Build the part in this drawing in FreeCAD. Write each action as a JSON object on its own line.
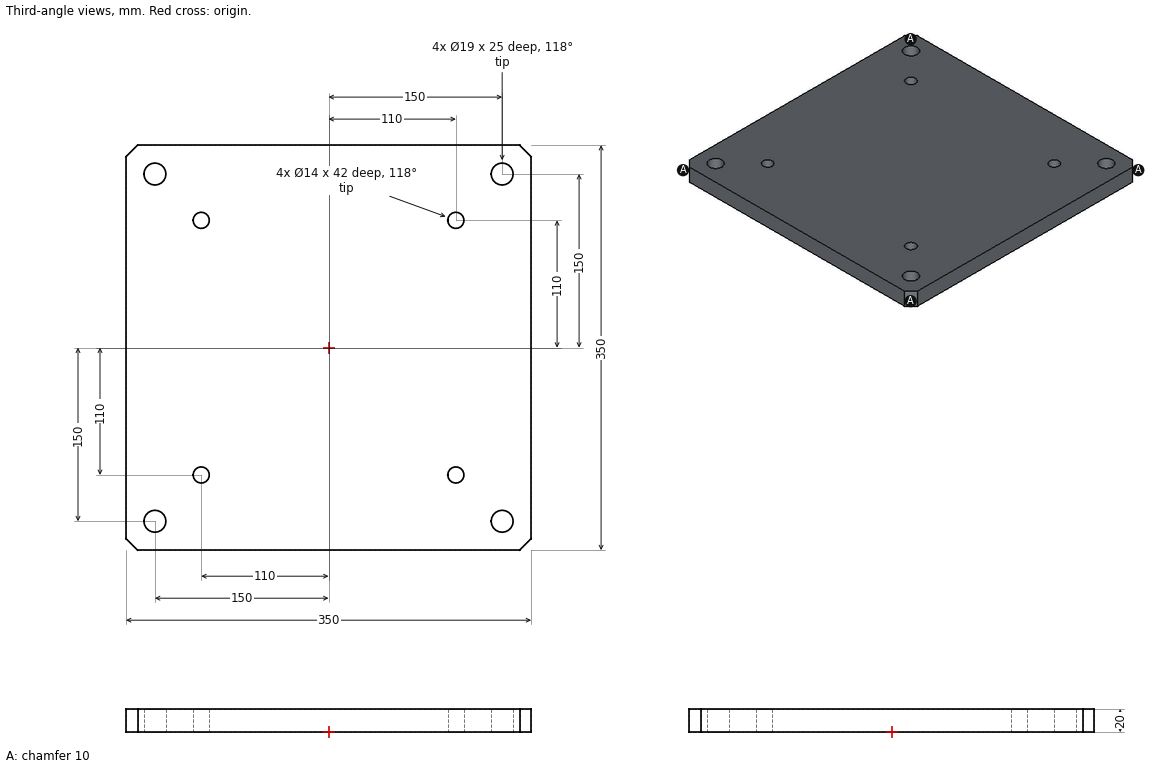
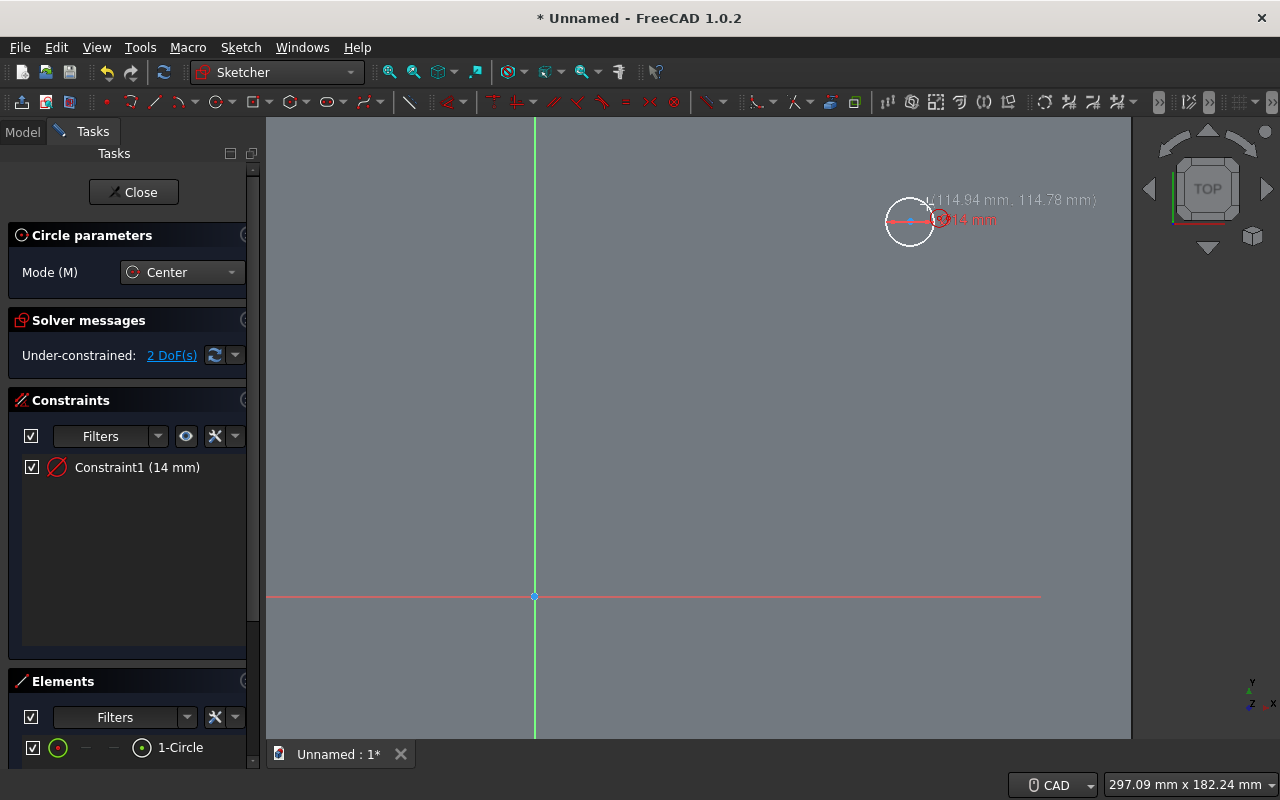
{"action": "scroll", "coordinate": [911, 223], "scroll_direction": "down", "scroll_amount": 3}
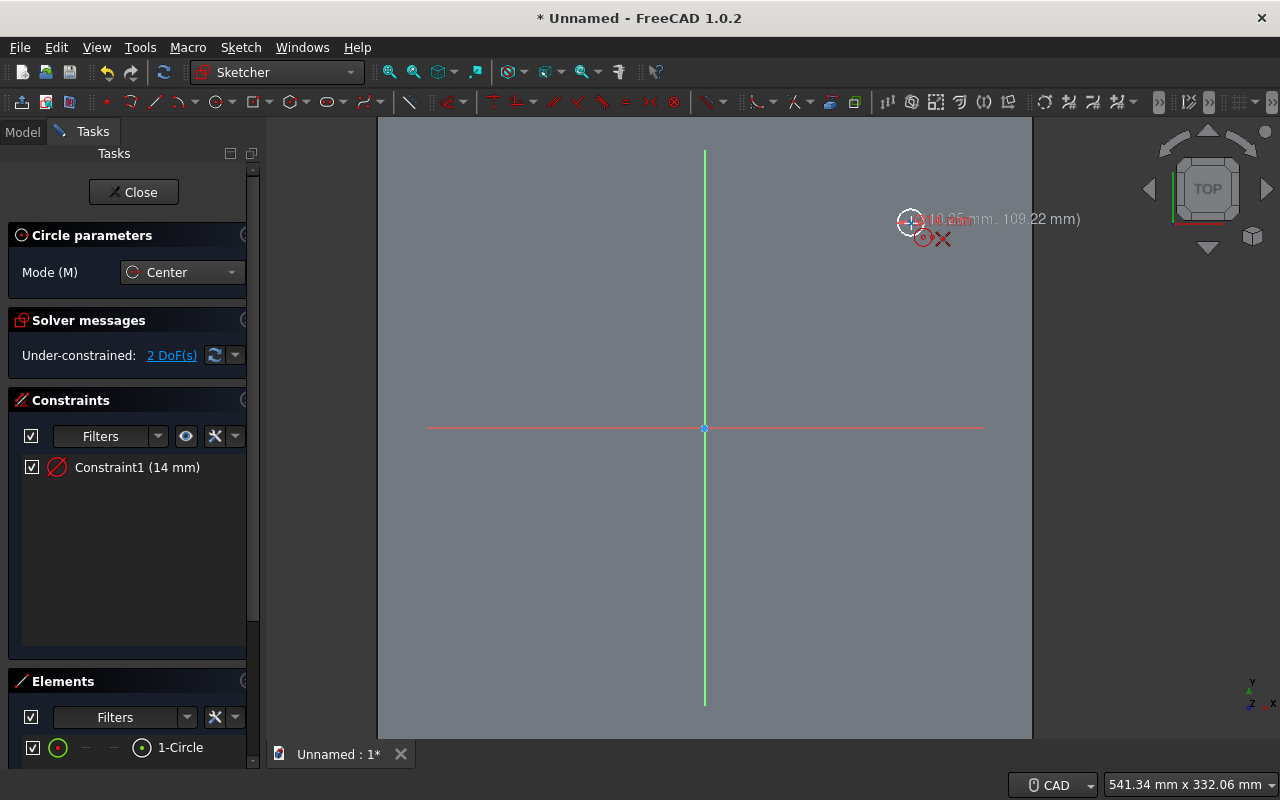
{"action": "scroll", "coordinate": [499, 634], "scroll_direction": "up", "scroll_amount": 3}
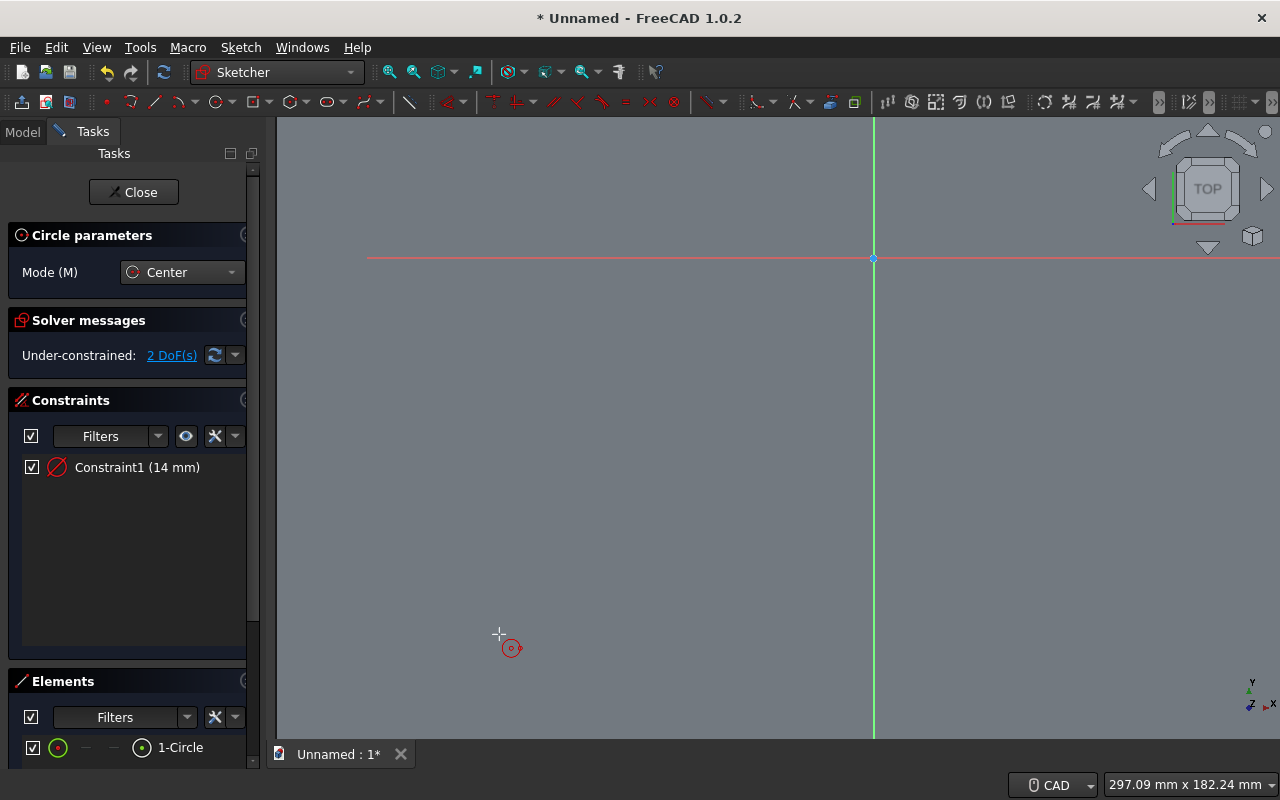
{"action": "left_click", "coordinate": [498, 634]}
{"action": "mouse_move", "coordinate": [515, 617]}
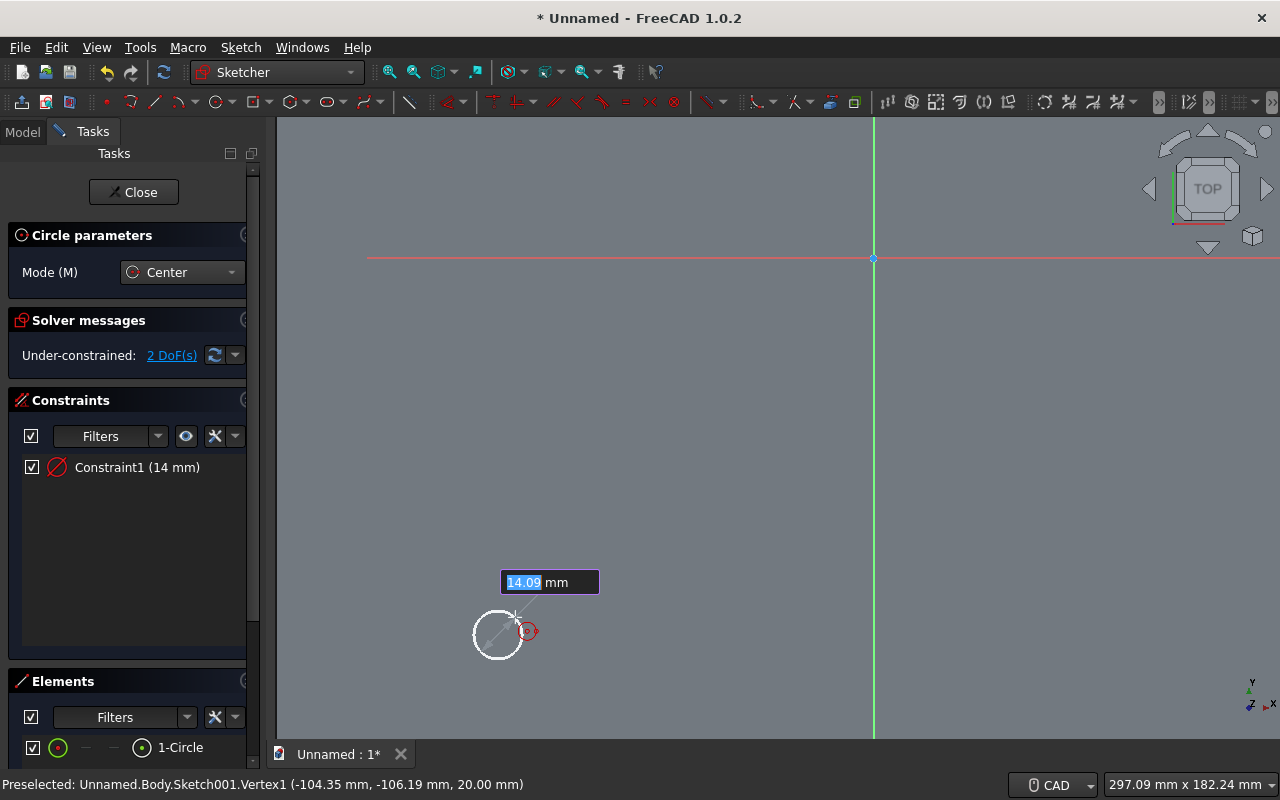
{"action": "type", "text": "14"}
{"action": "key", "text": "Return"}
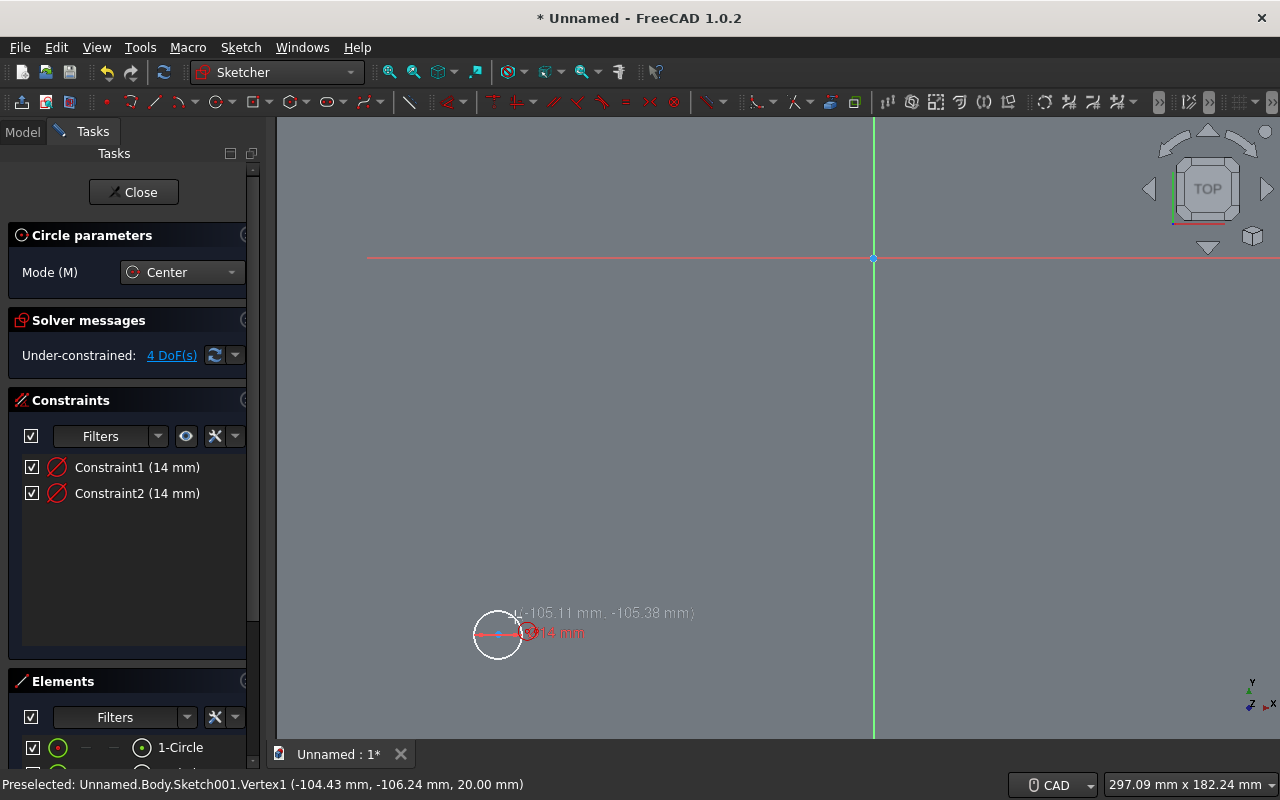
{"action": "scroll", "coordinate": [499, 634], "scroll_direction": "down", "scroll_amount": 3}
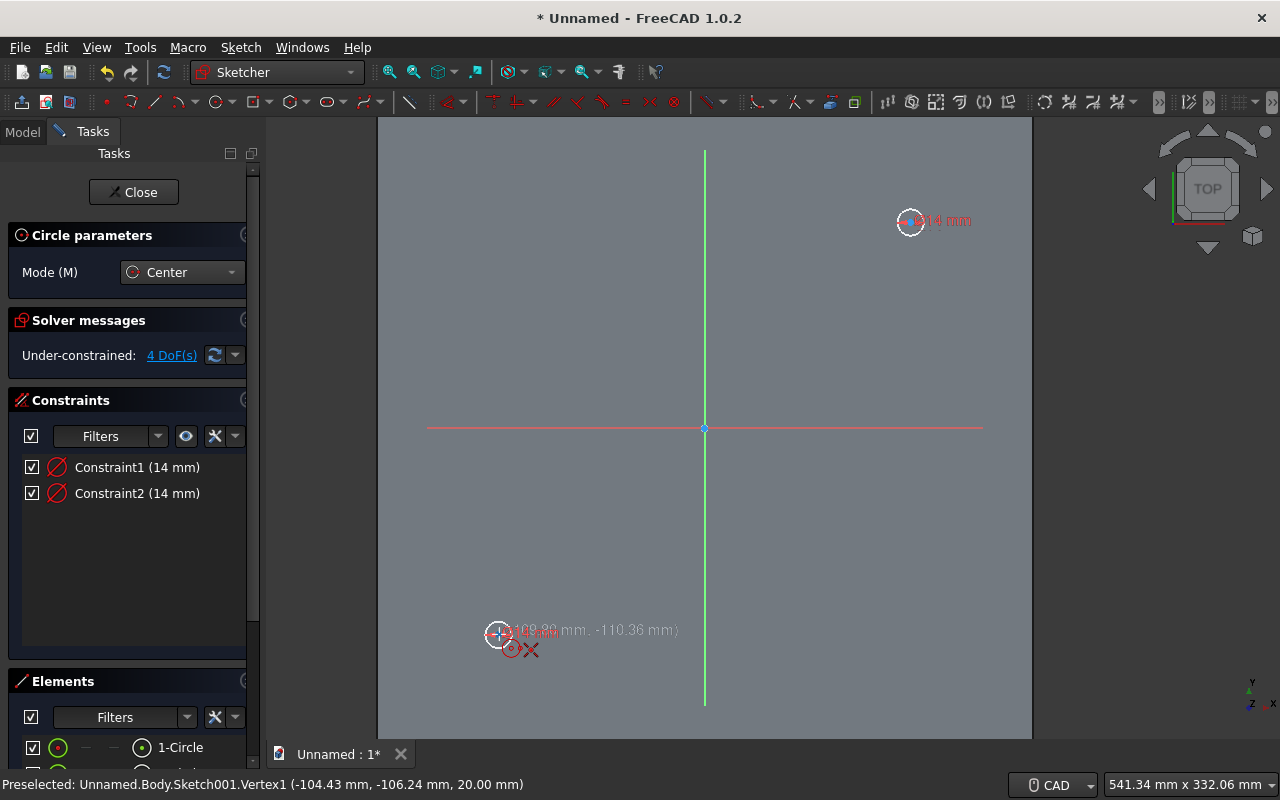
{"action": "scroll", "coordinate": [499, 222], "scroll_direction": "up", "scroll_amount": 3}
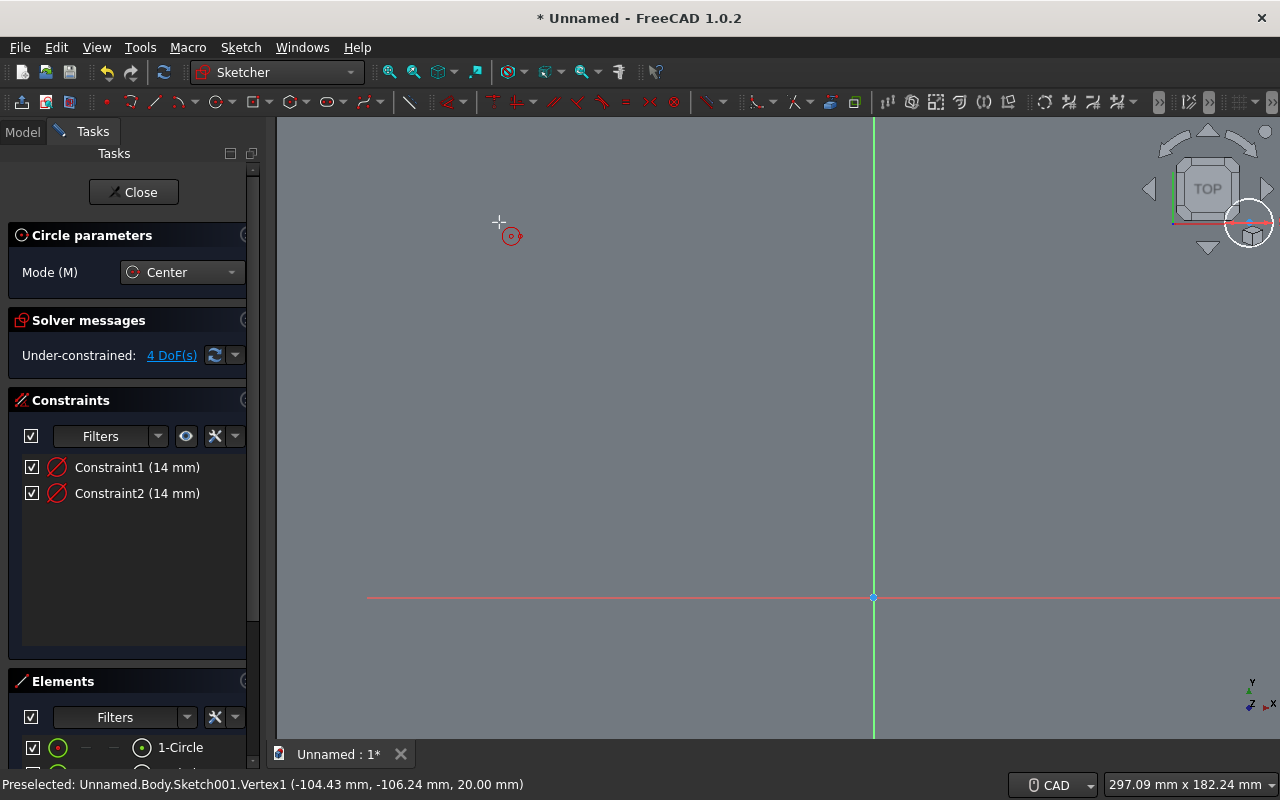
{"action": "left_click", "coordinate": [498, 222]}
{"action": "mouse_move", "coordinate": [515, 205]}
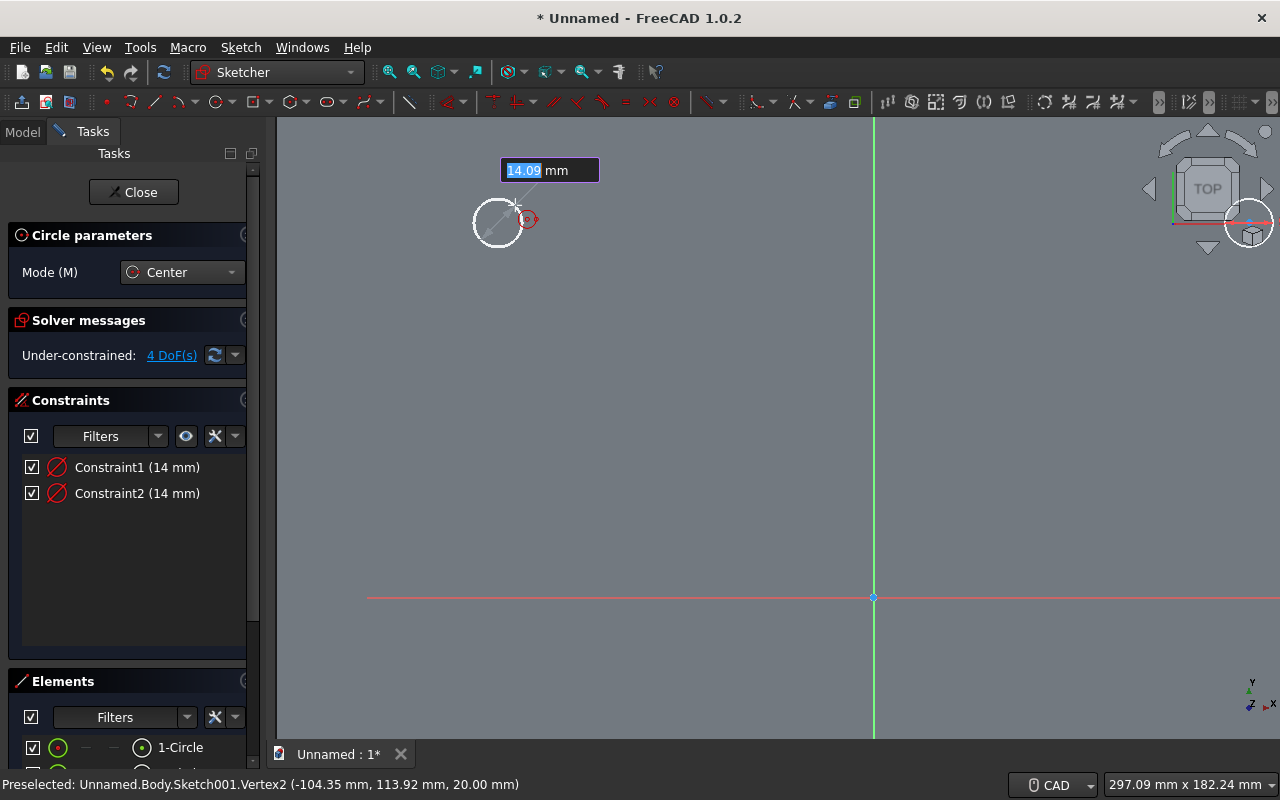
{"action": "type", "text": "14"}
{"action": "key", "text": "Return"}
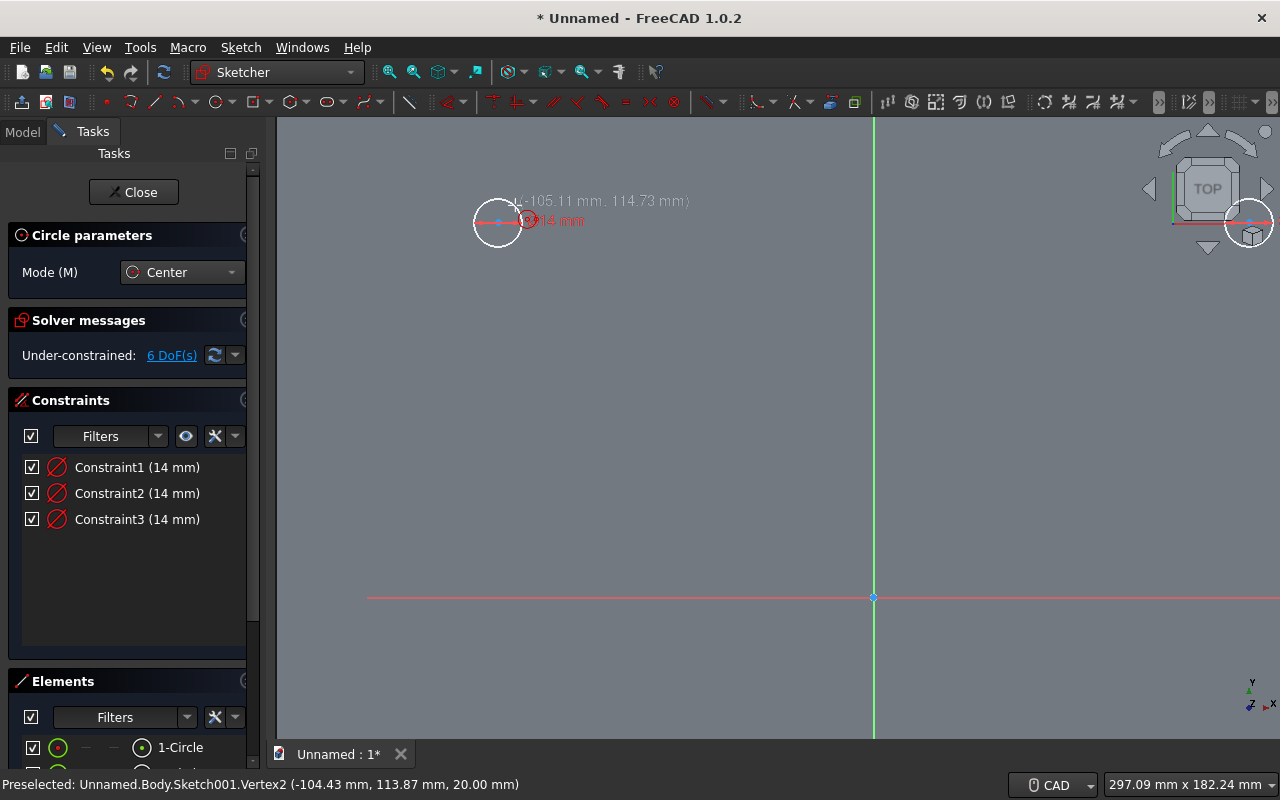
{"action": "scroll", "coordinate": [499, 222], "scroll_direction": "down", "scroll_amount": 3}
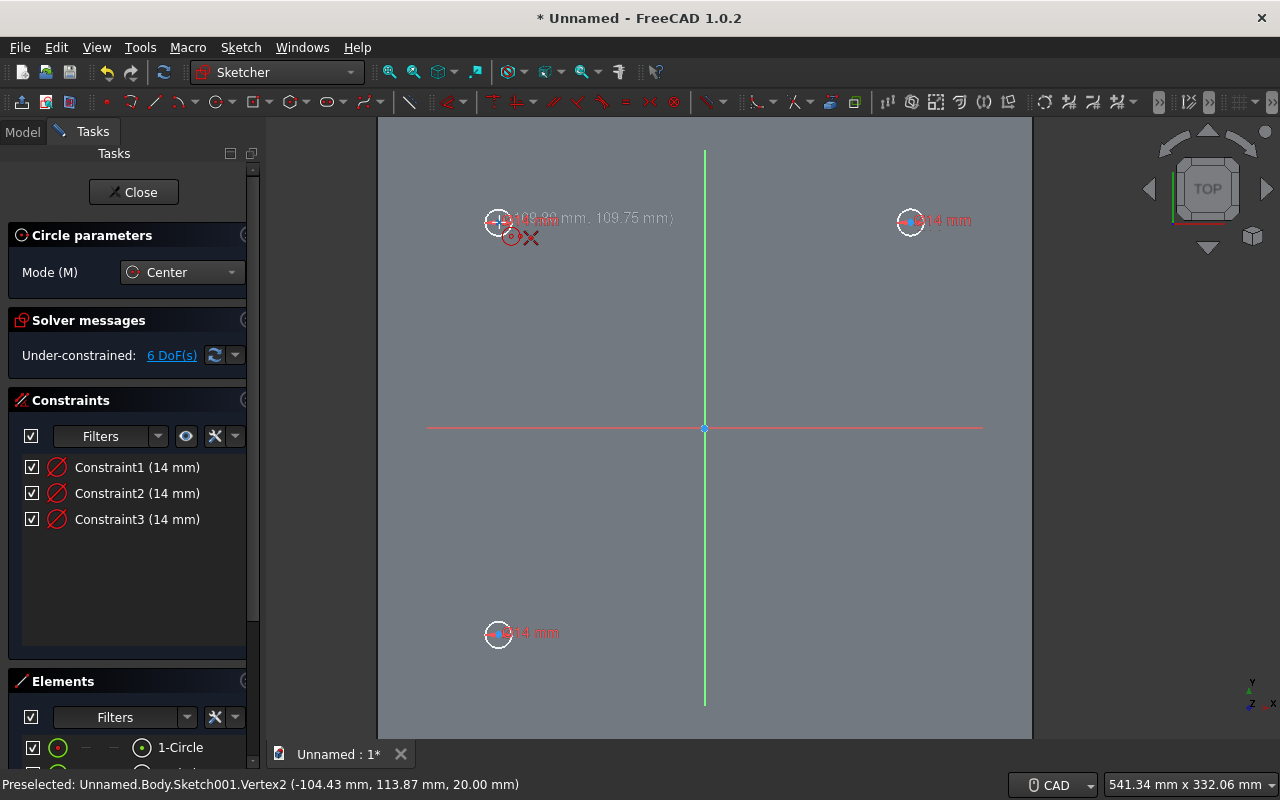
{"action": "scroll", "coordinate": [911, 634], "scroll_direction": "up", "scroll_amount": 3}